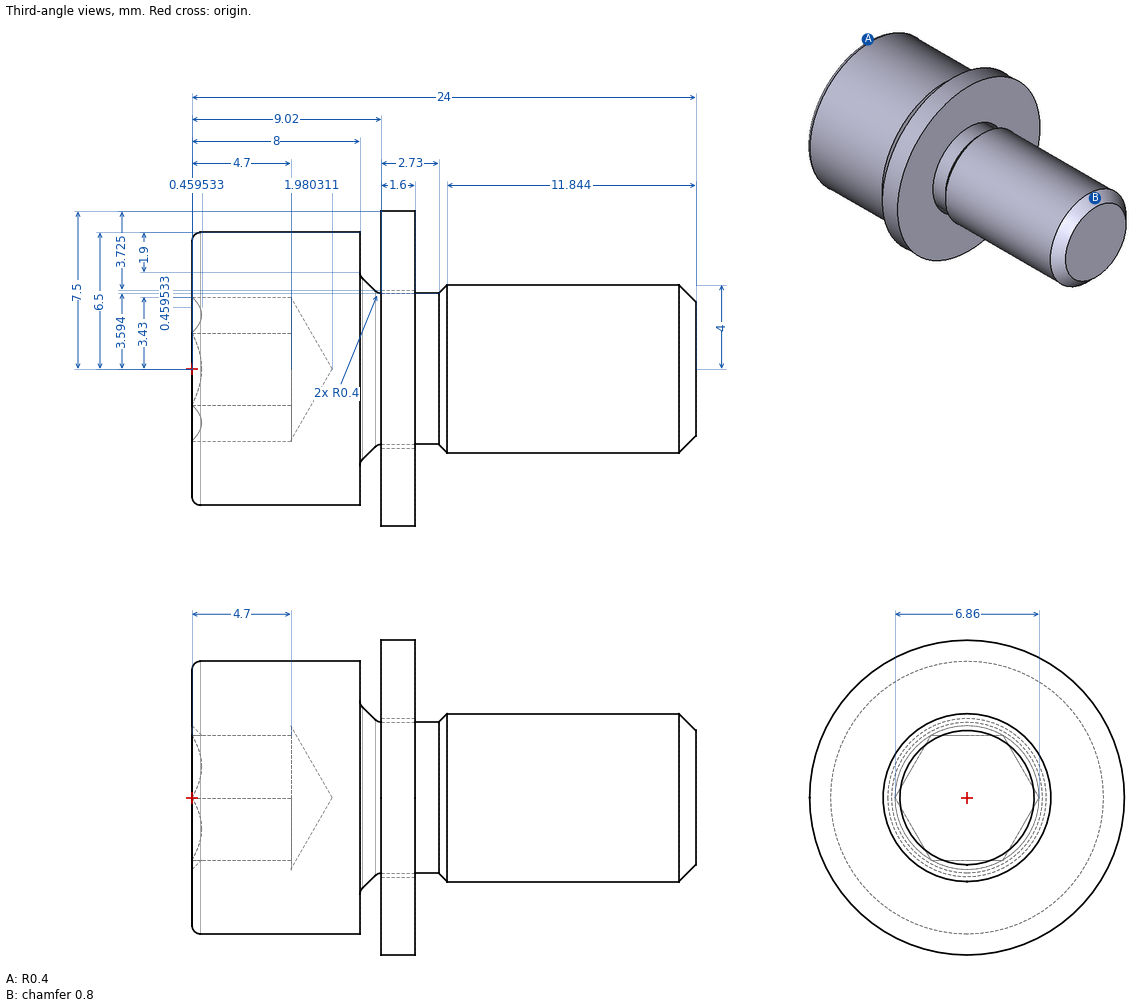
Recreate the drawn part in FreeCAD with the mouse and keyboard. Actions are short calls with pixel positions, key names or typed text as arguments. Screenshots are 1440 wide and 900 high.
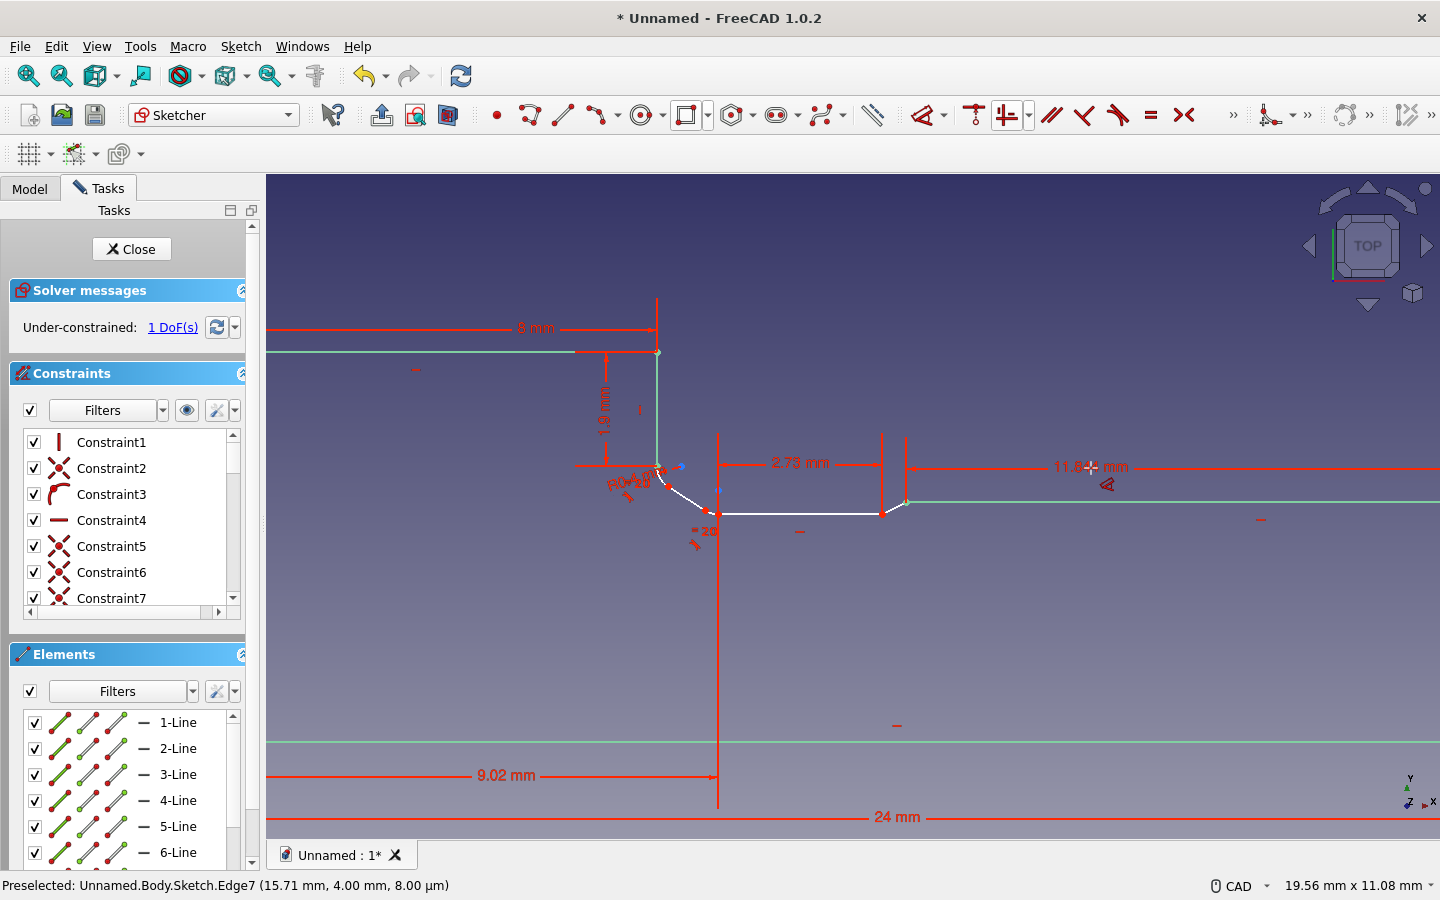
click(882, 514)
click(916, 628)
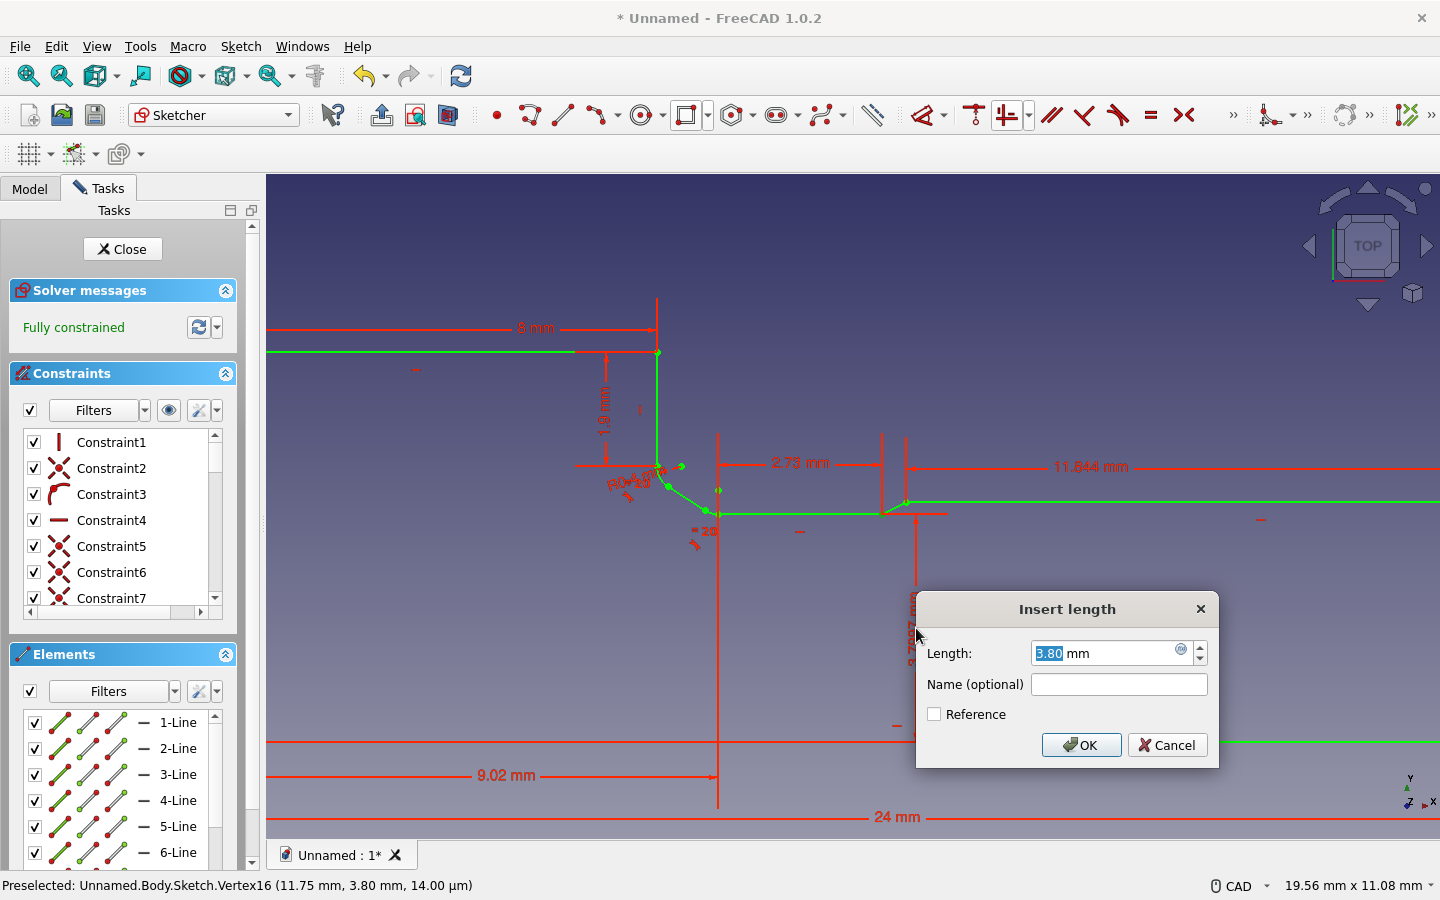
text(3.594)
key(Return)
key(Escape)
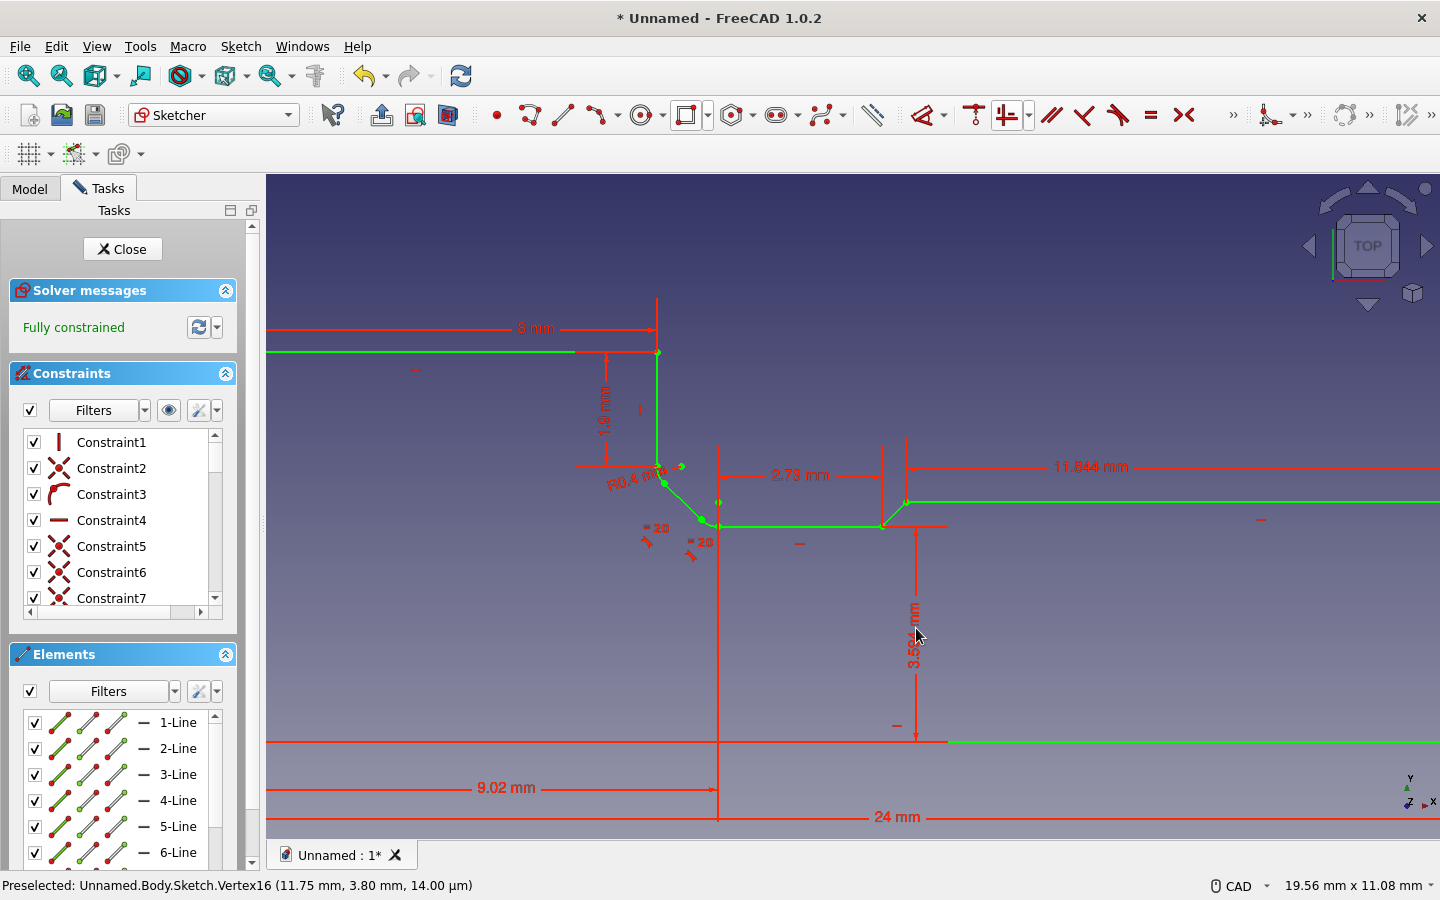
click(123, 249)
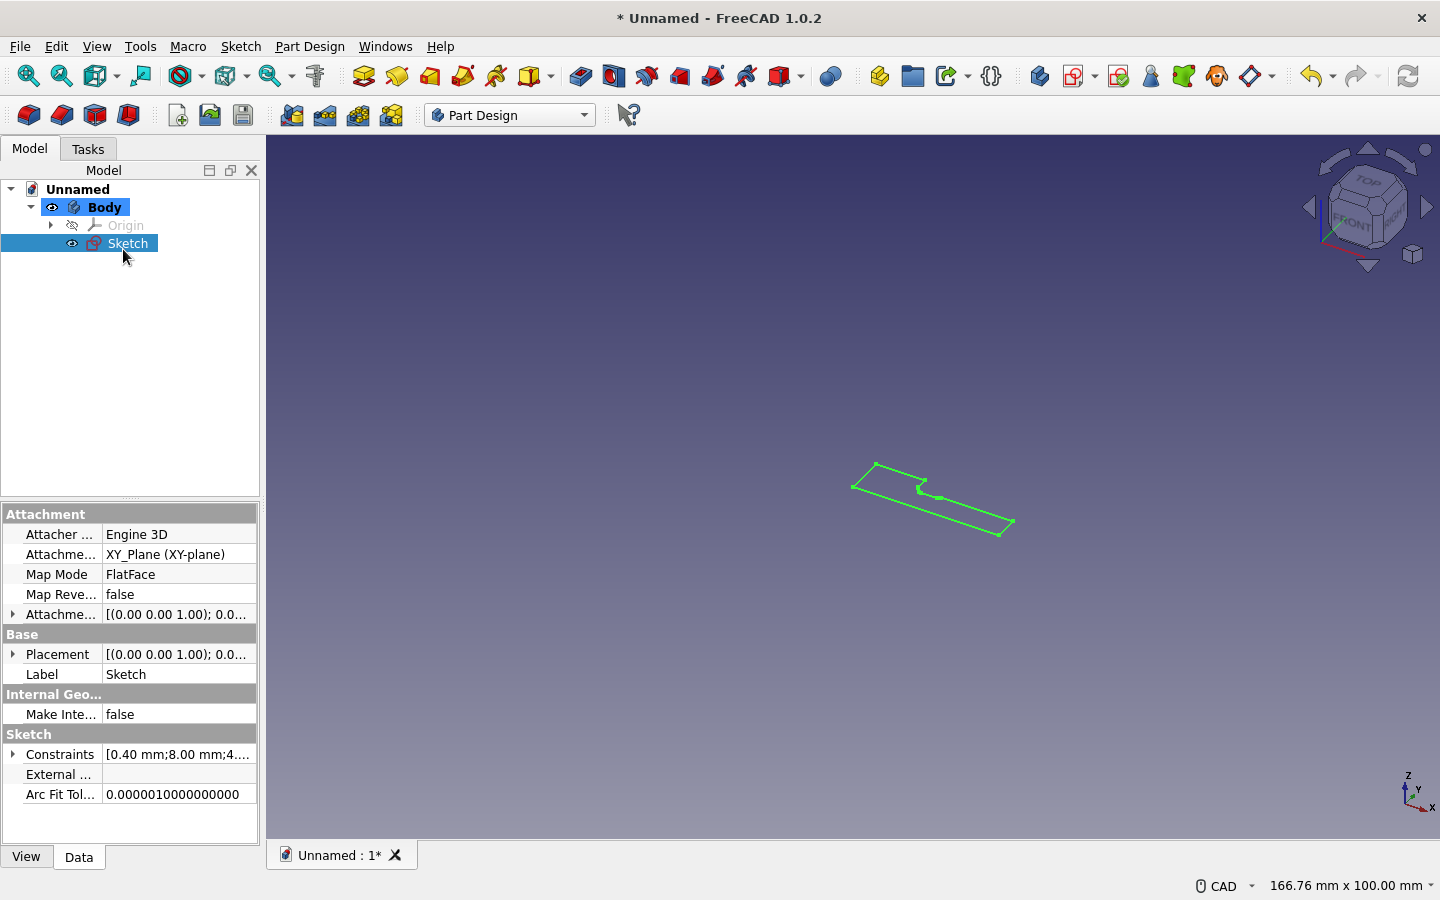
click(397, 76)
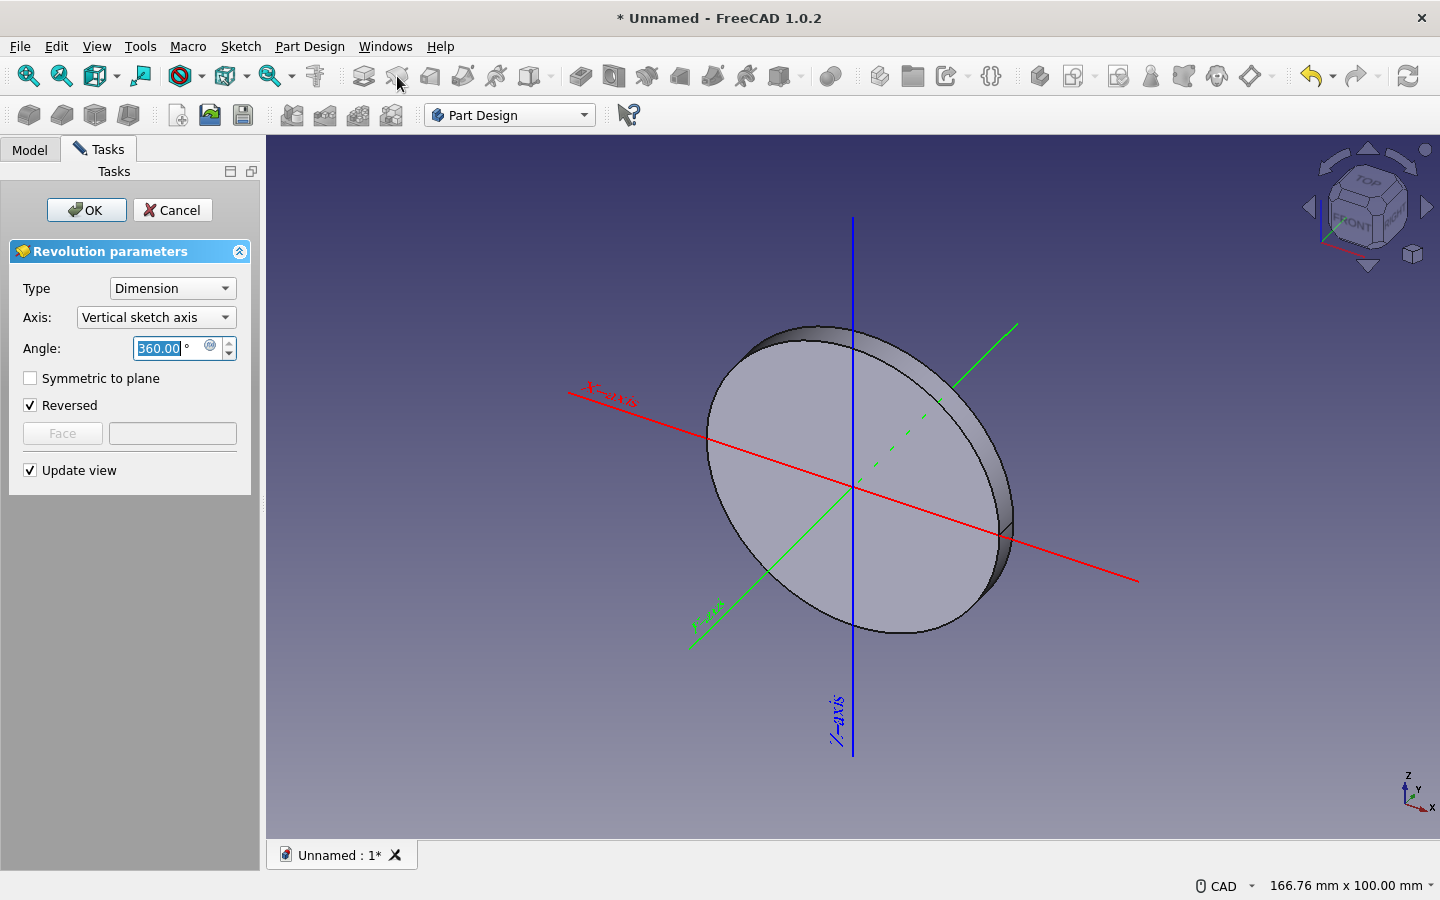
click(157, 318)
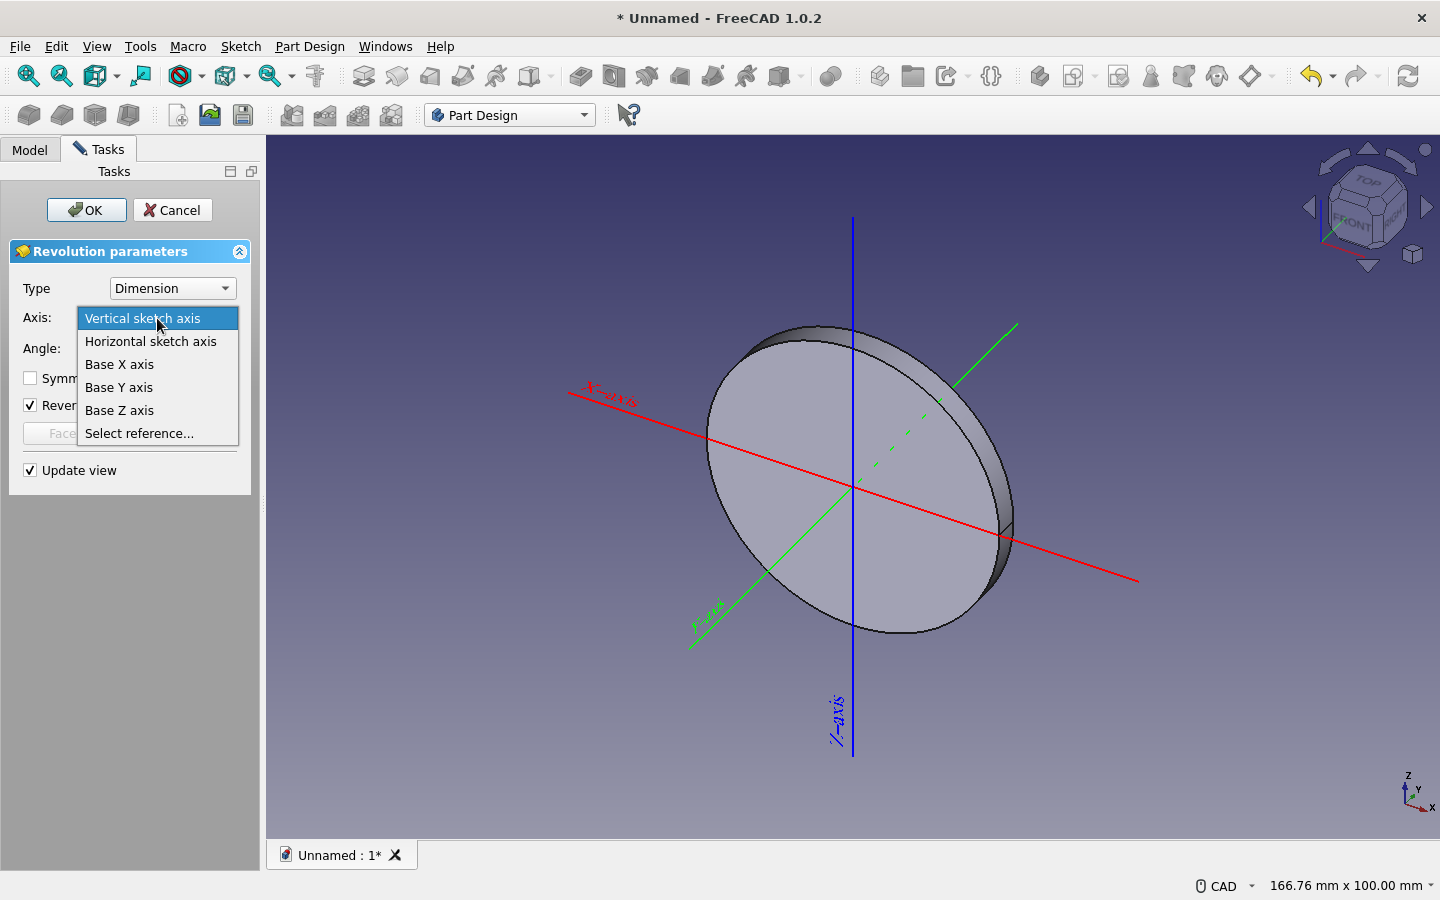
click(156, 342)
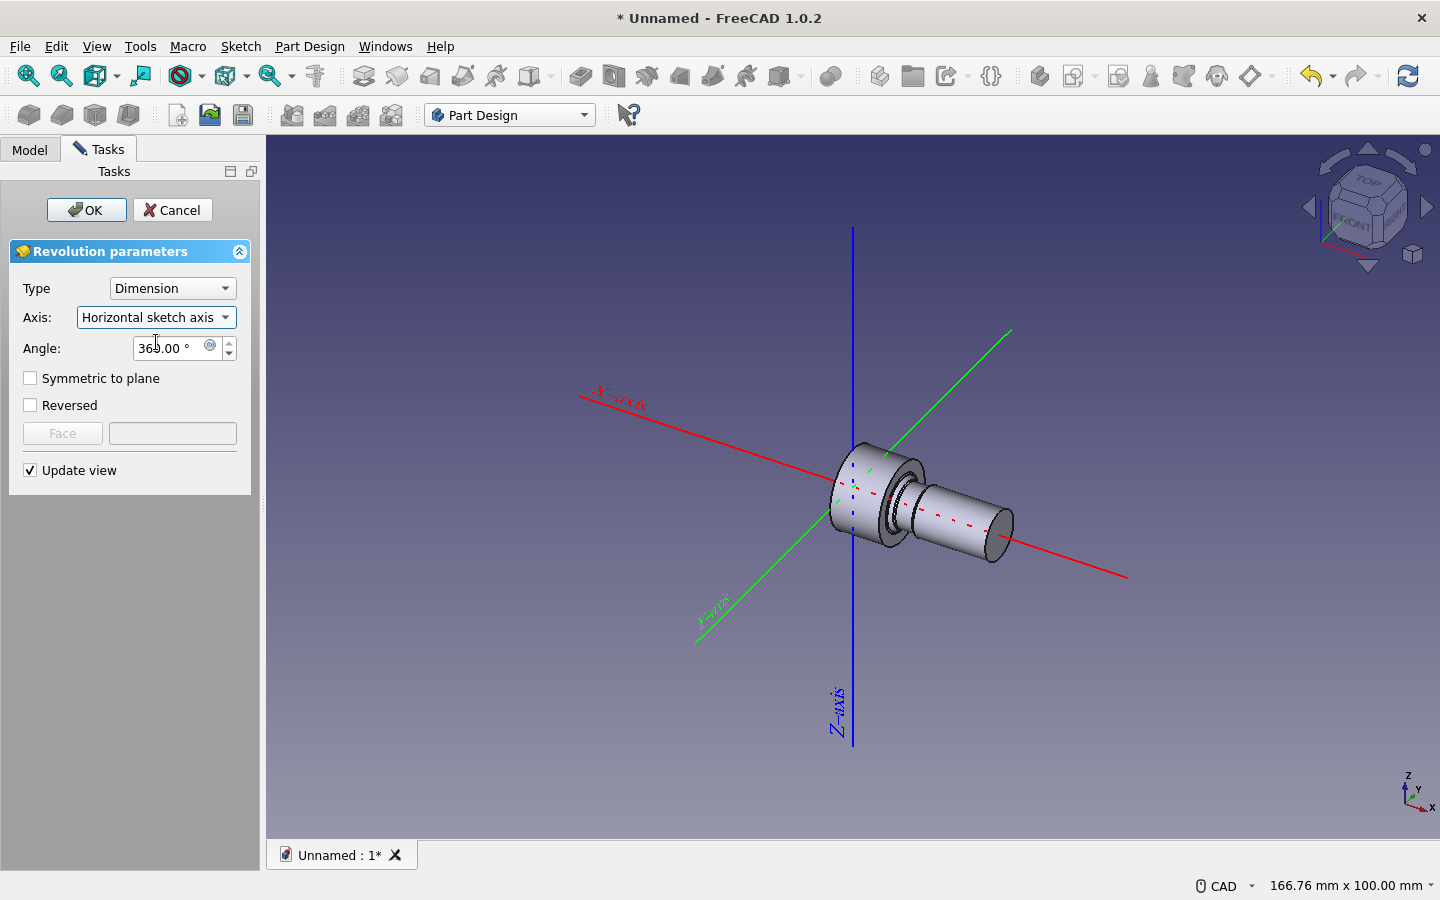
click(87, 210)